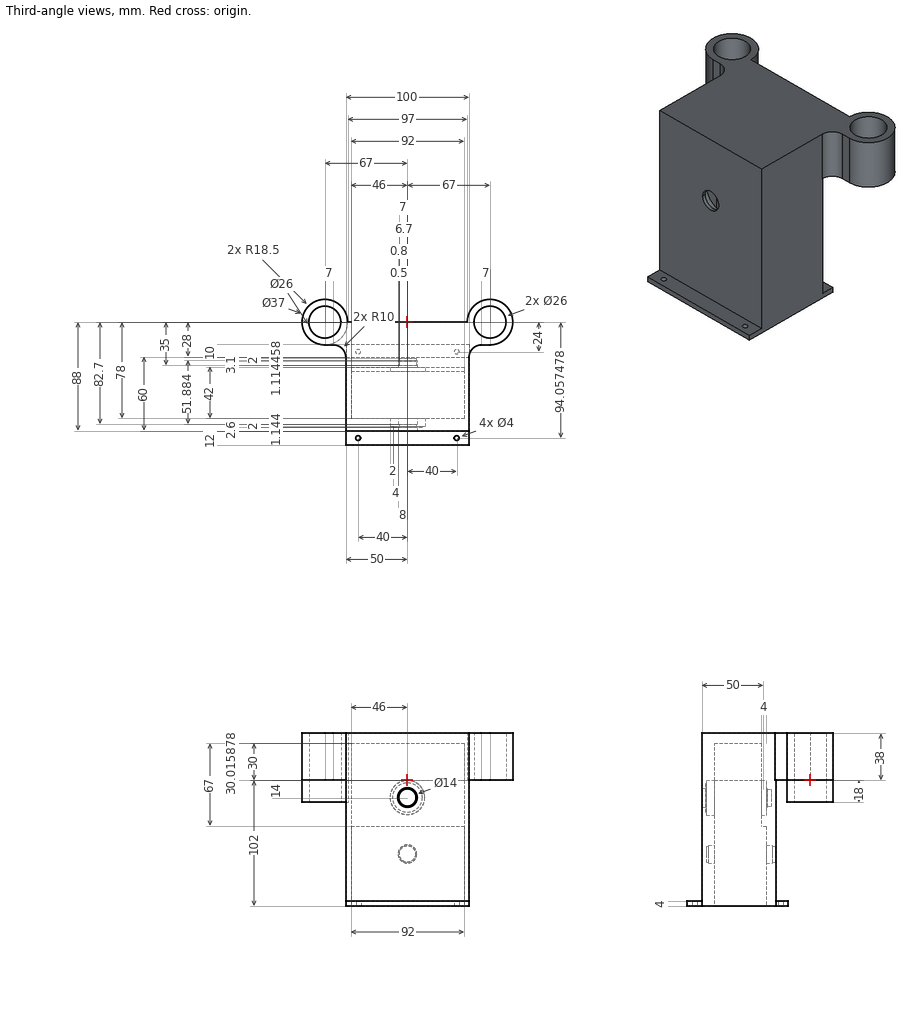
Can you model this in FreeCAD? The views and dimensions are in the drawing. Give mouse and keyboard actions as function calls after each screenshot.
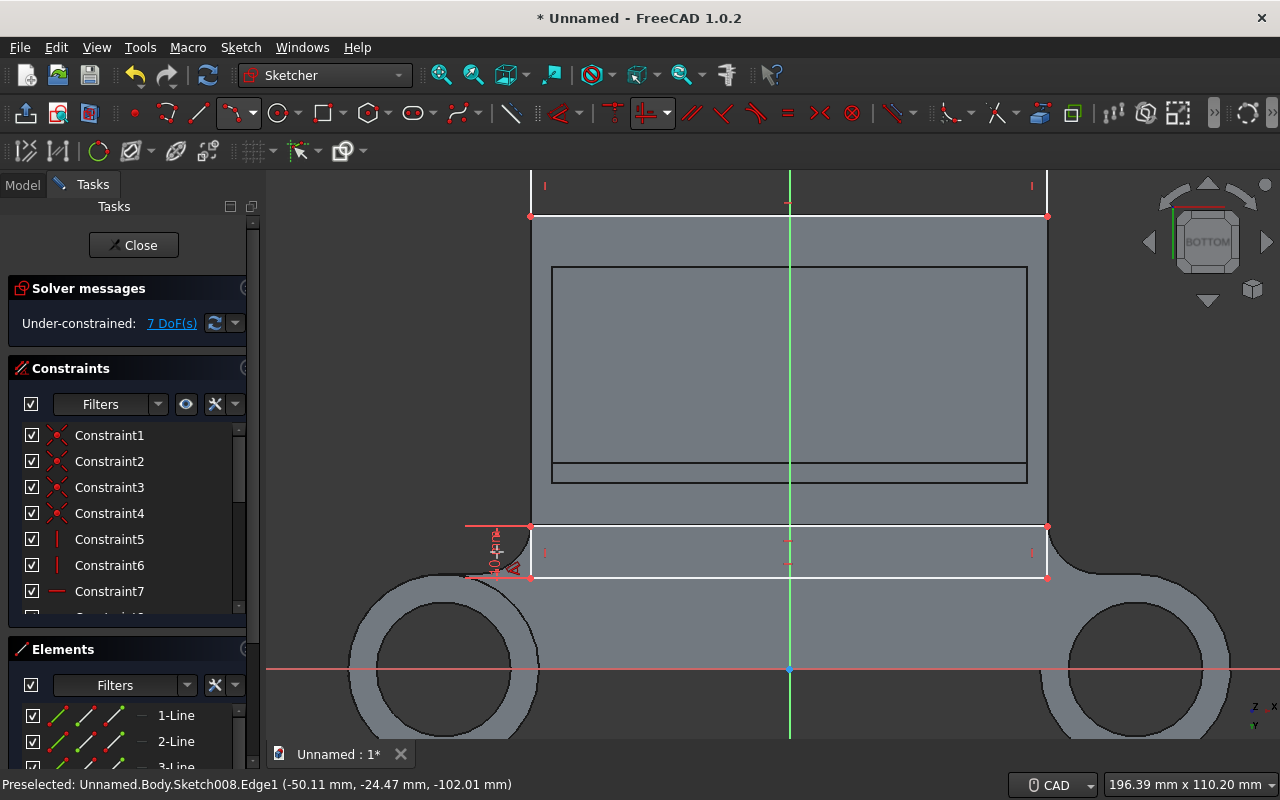
click(531, 204)
click(497, 207)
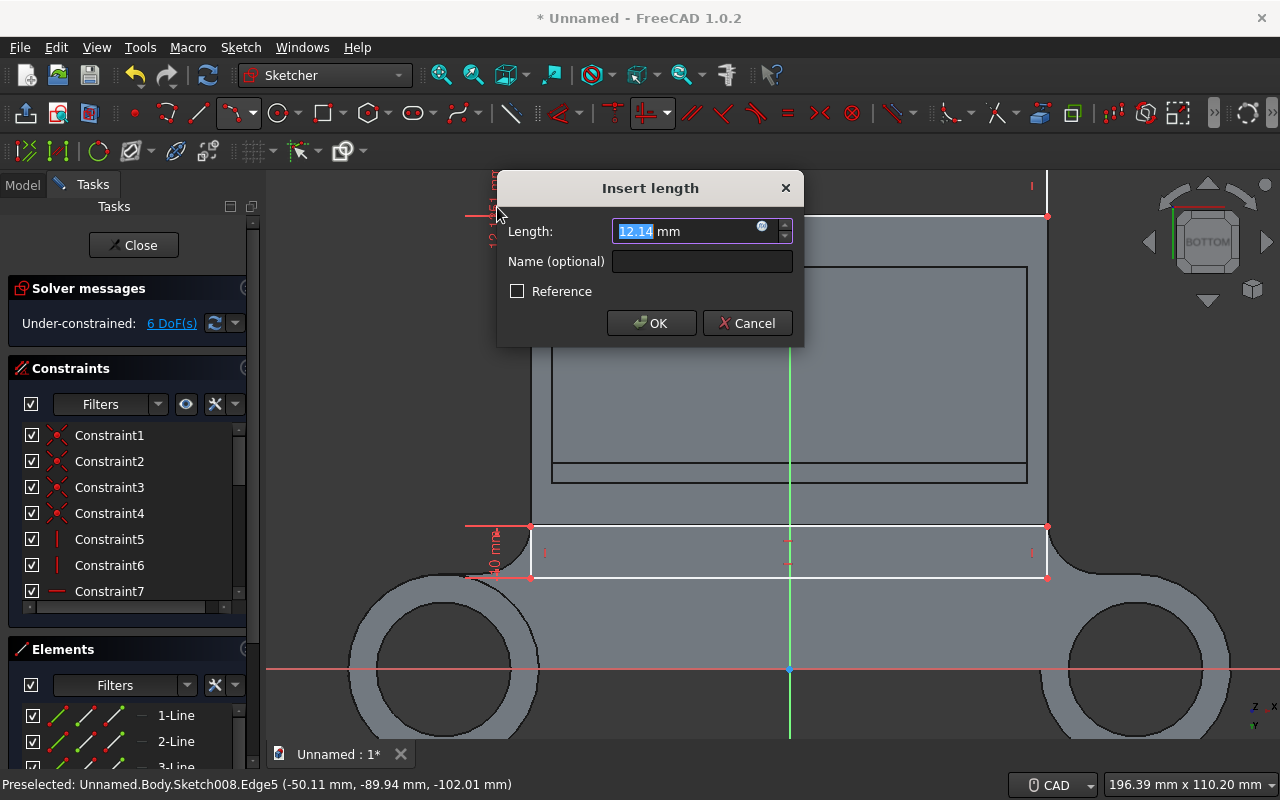
text(12)
key(Return)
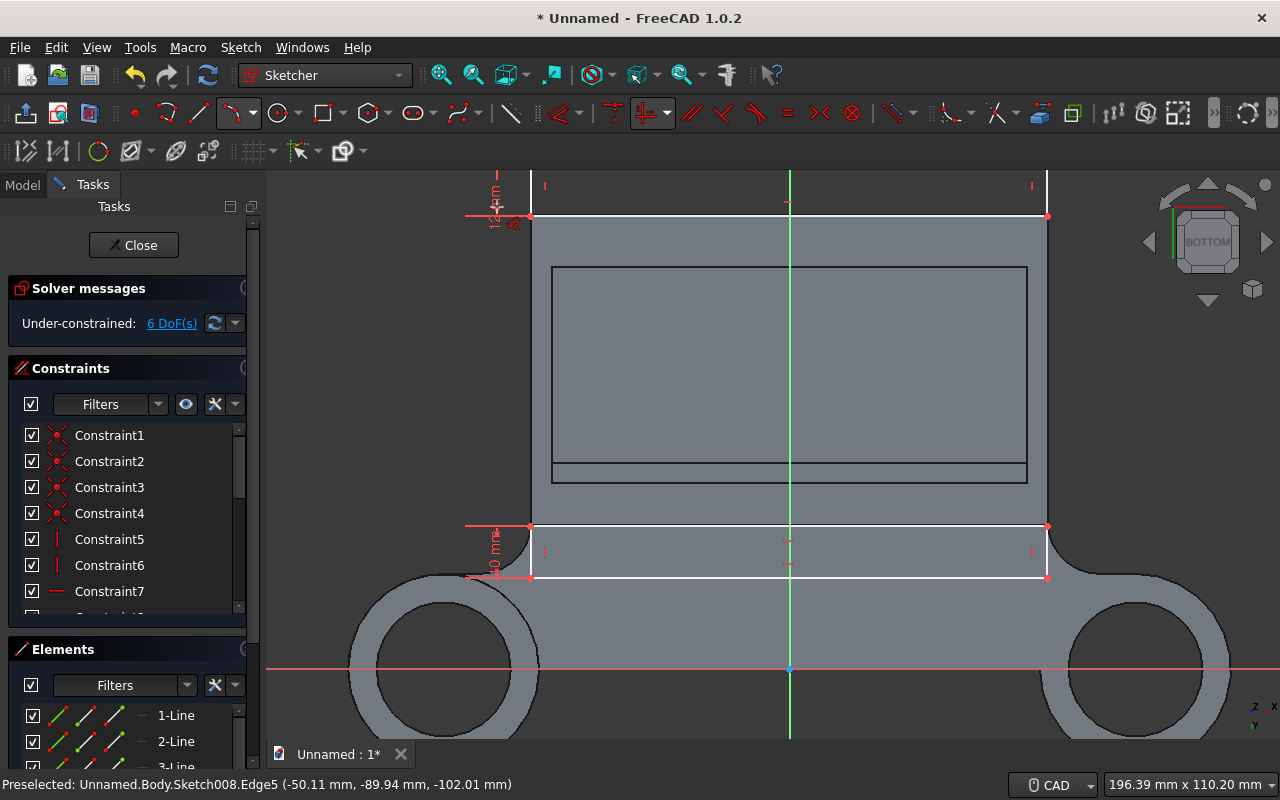
click(686, 578)
click(670, 612)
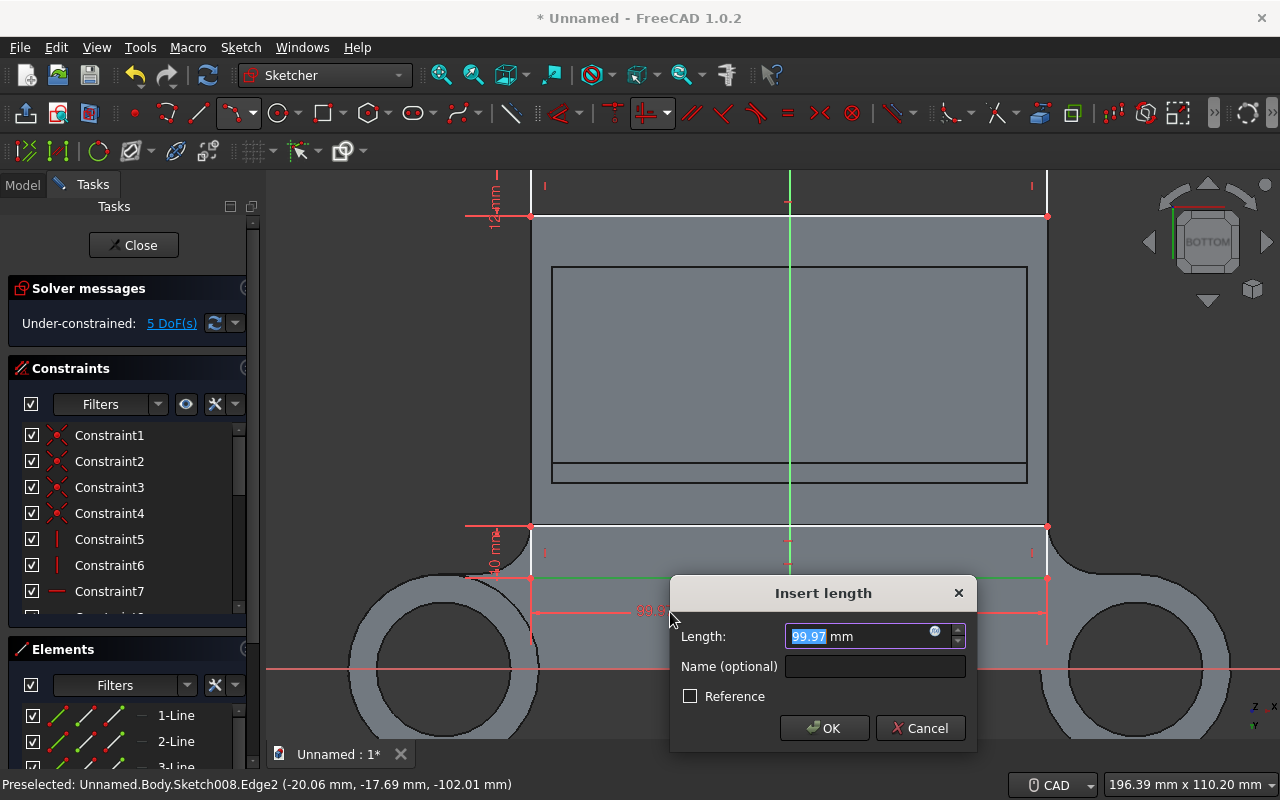
text(100)
key(Return)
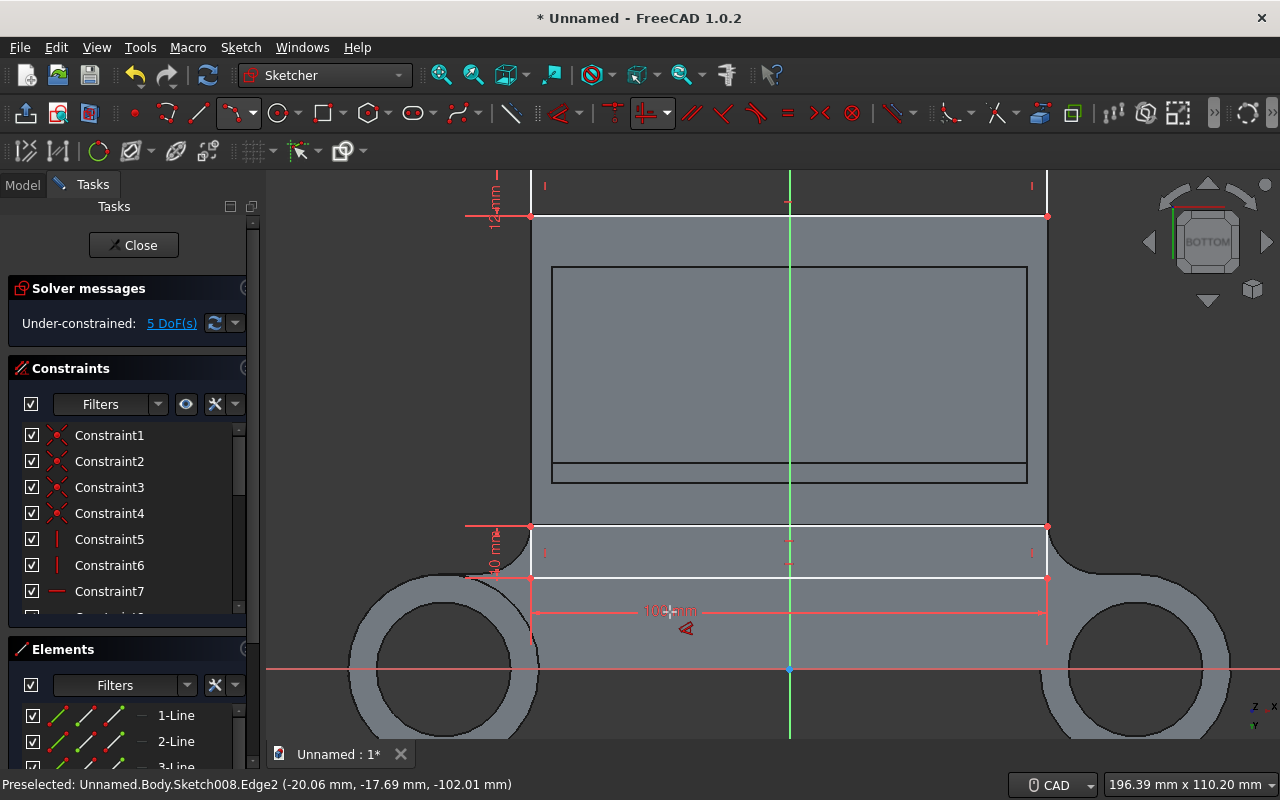
click(686, 216)
click(670, 250)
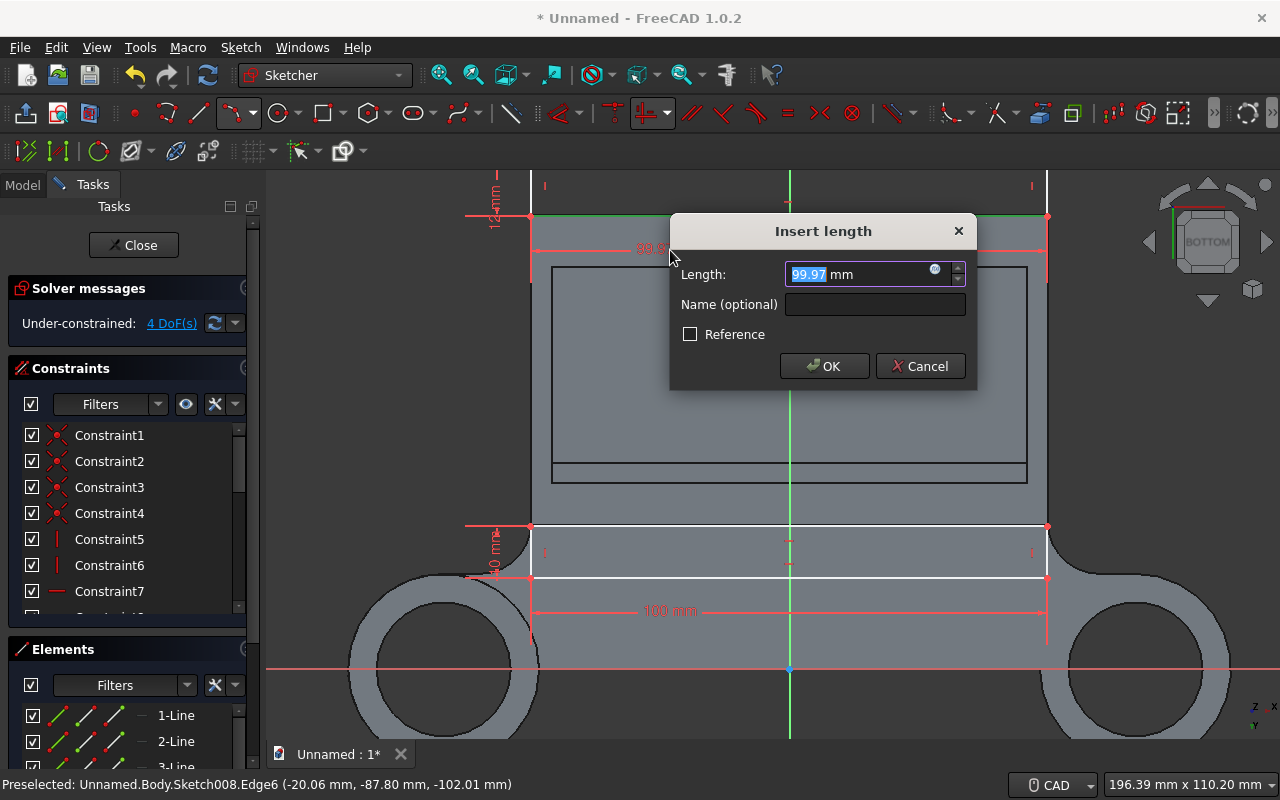
text(100)
key(Return)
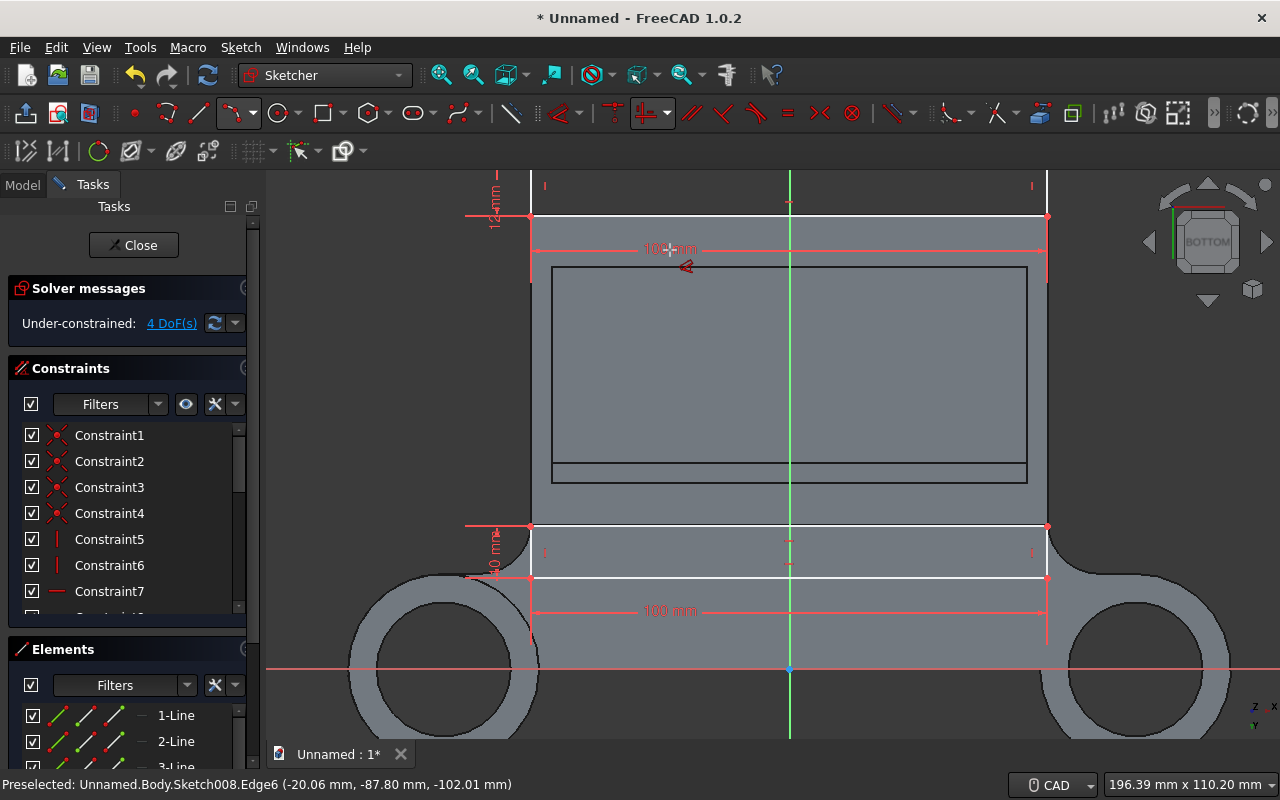
click(531, 526)
click(660, 703)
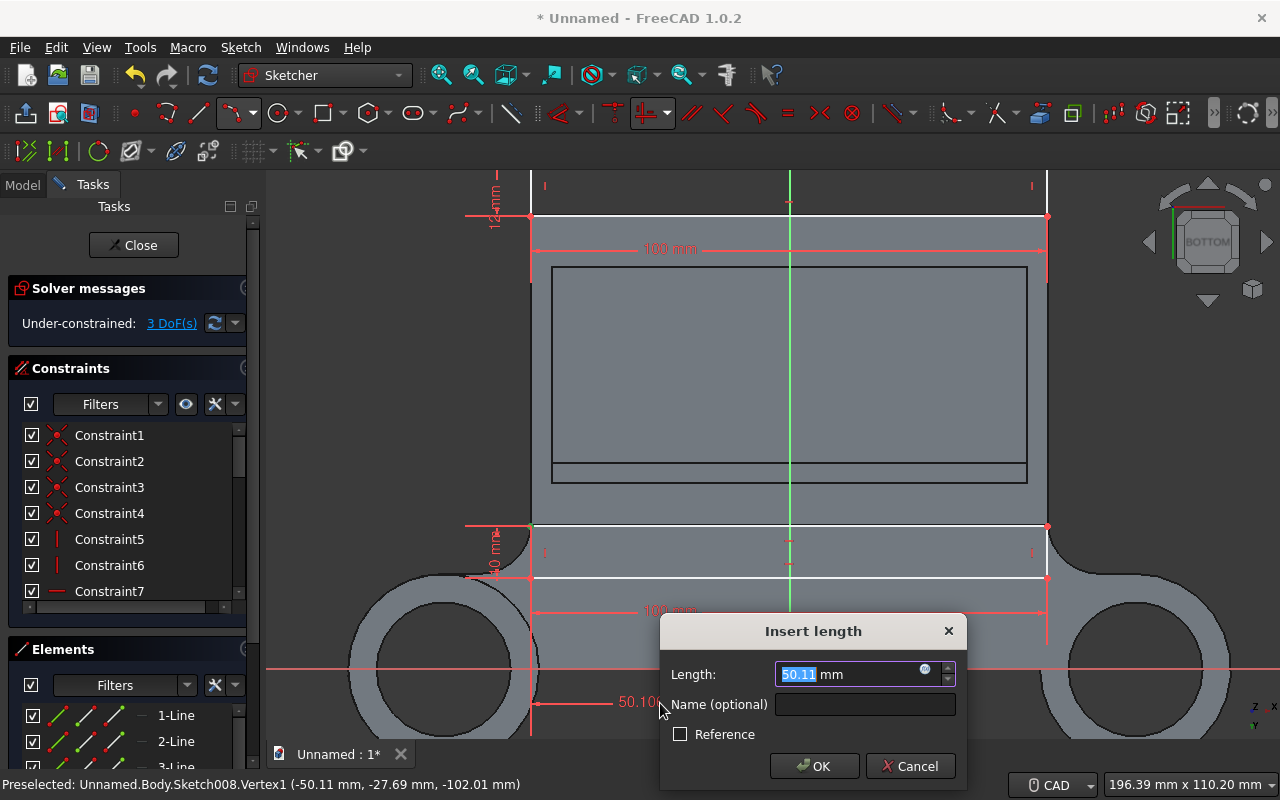
text(50)
key(Return)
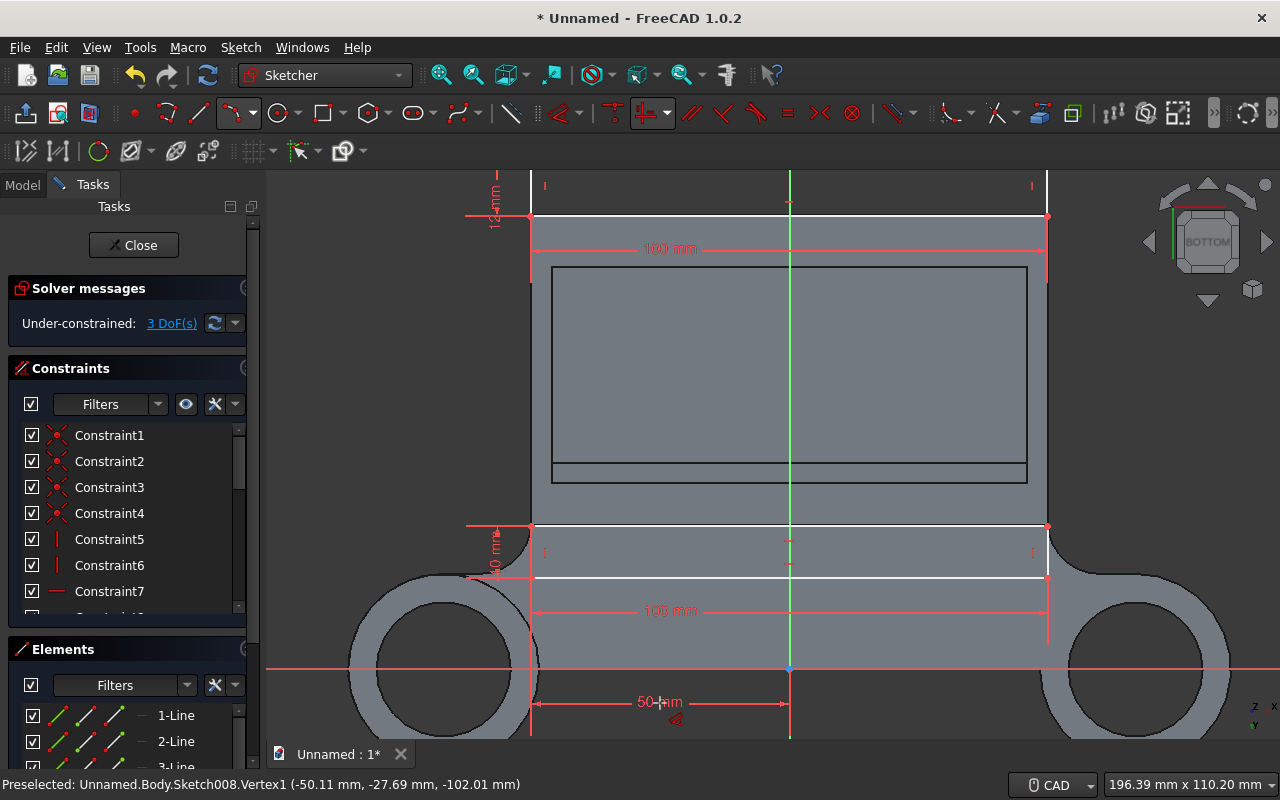
click(531, 526)
click(497, 598)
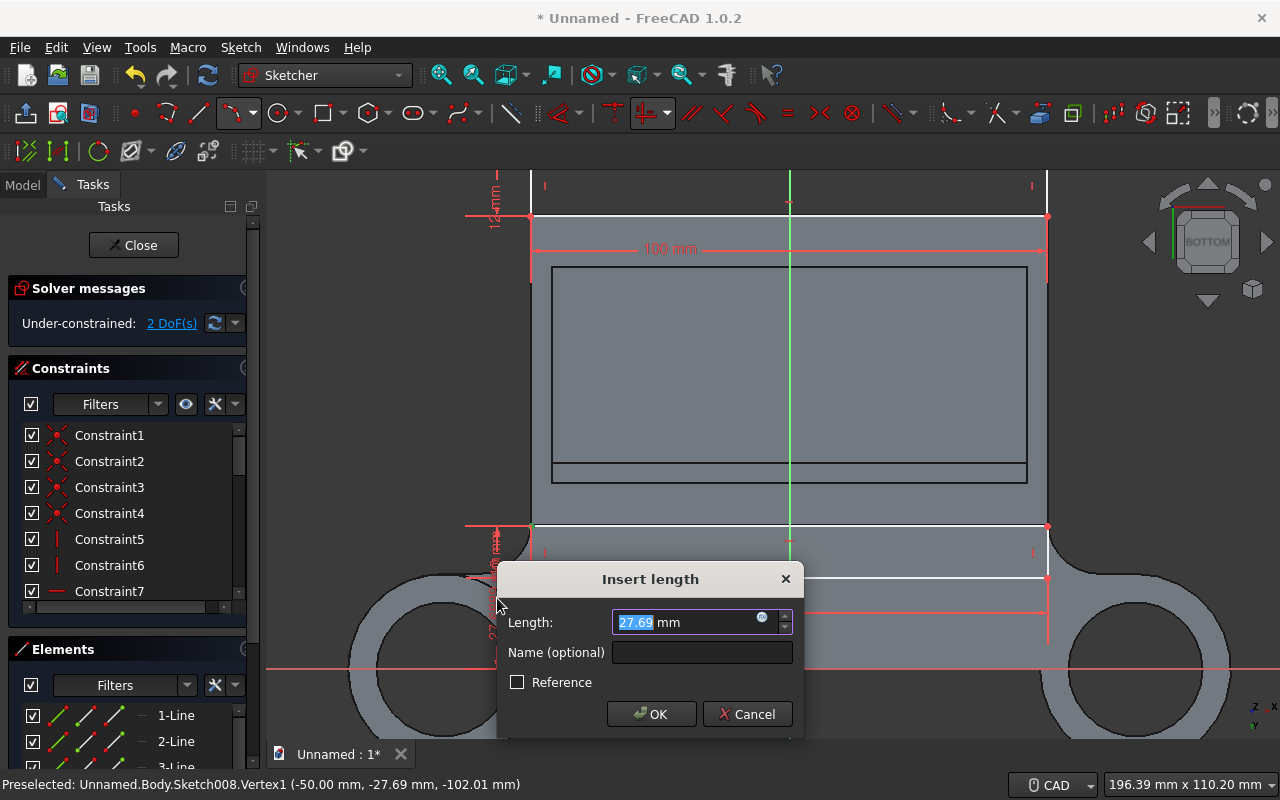
text(28)
key(Return)